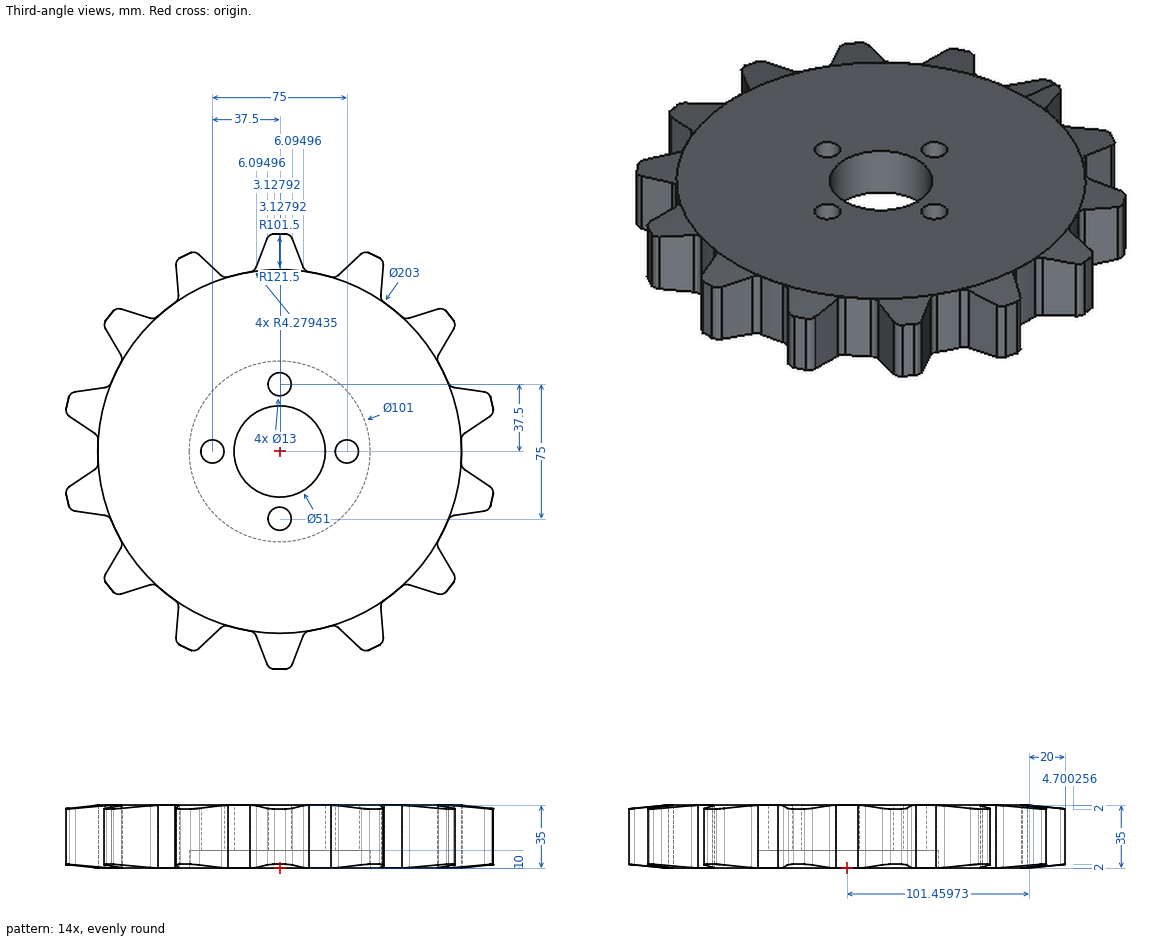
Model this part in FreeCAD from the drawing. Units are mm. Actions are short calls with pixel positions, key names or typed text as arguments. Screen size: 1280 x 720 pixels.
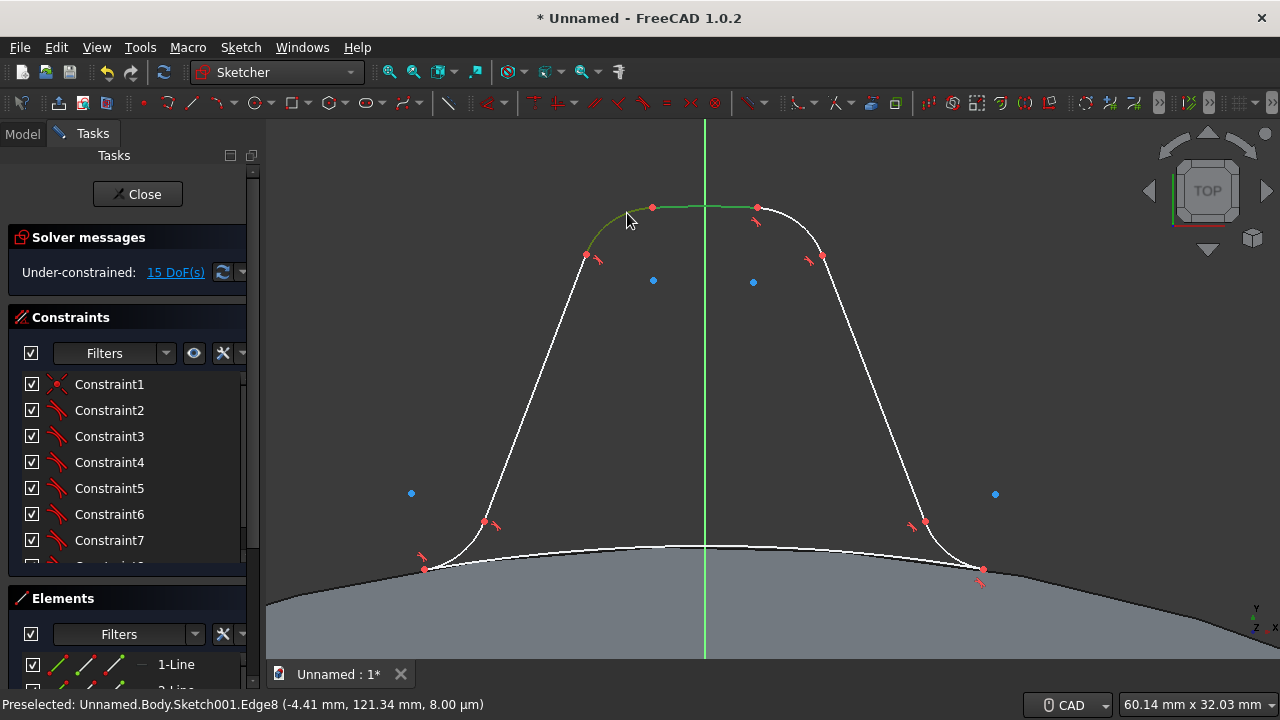
click(644, 104)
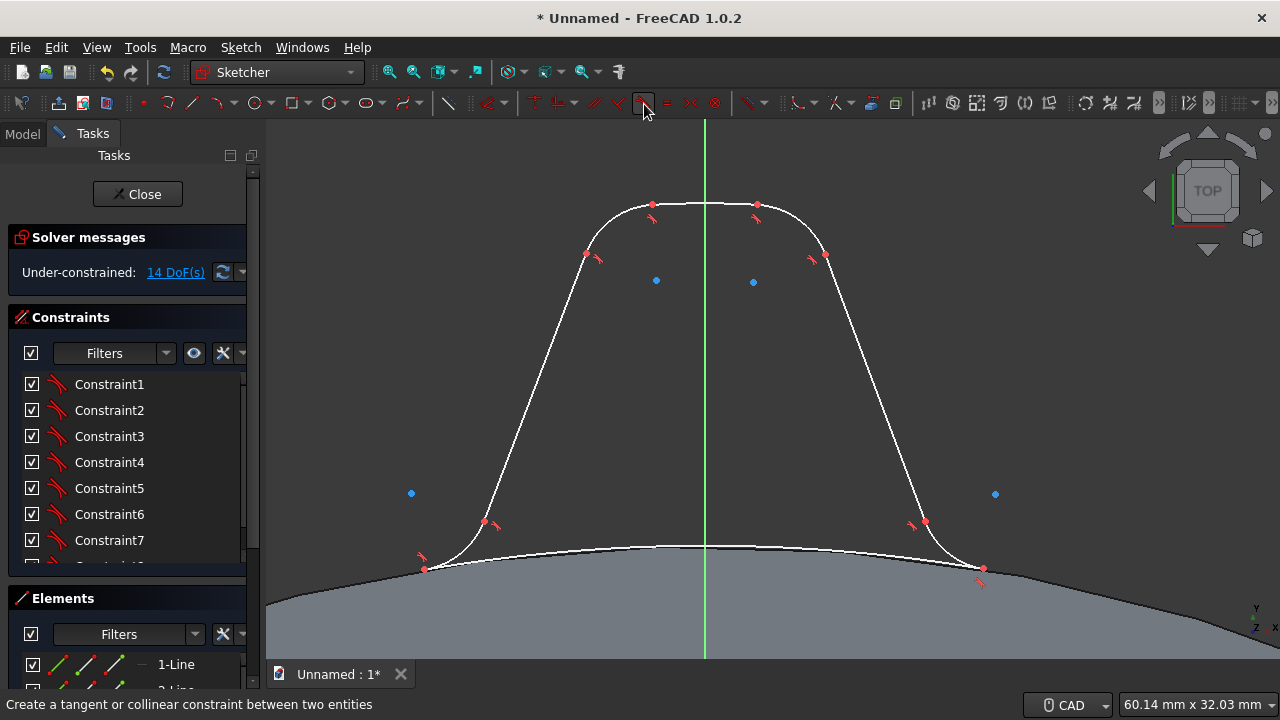
click(816, 549)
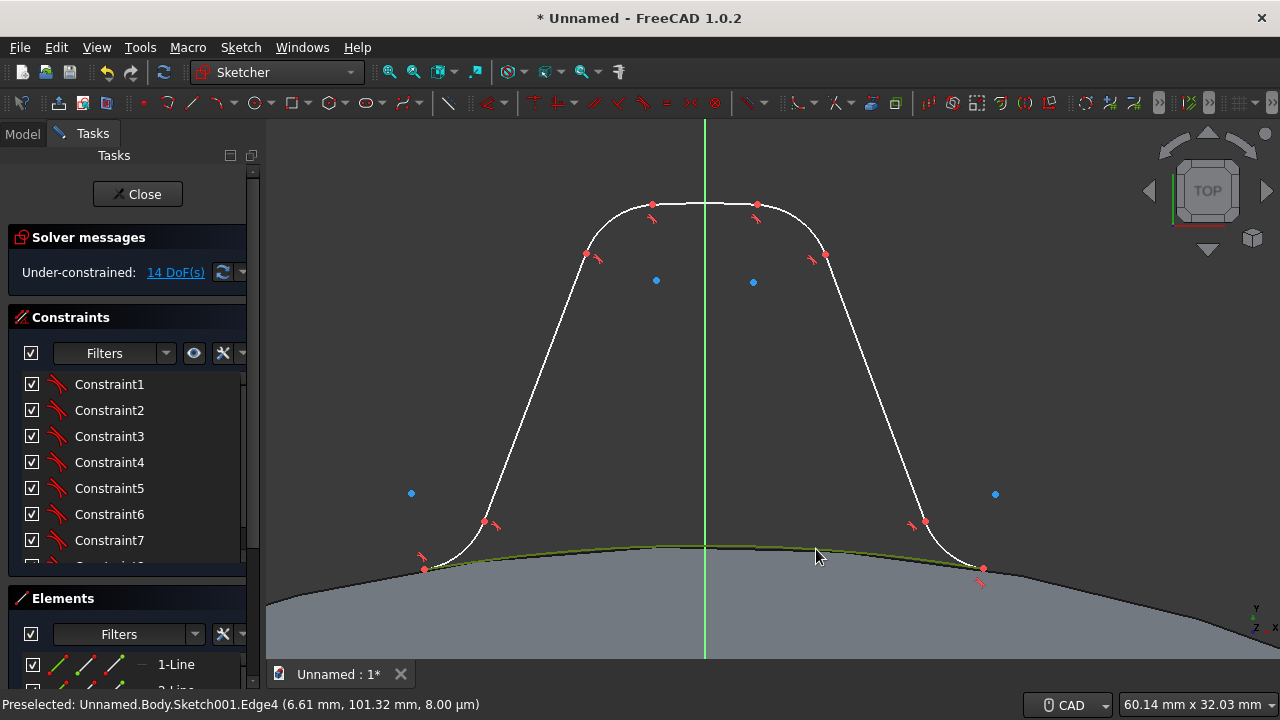
click(726, 204)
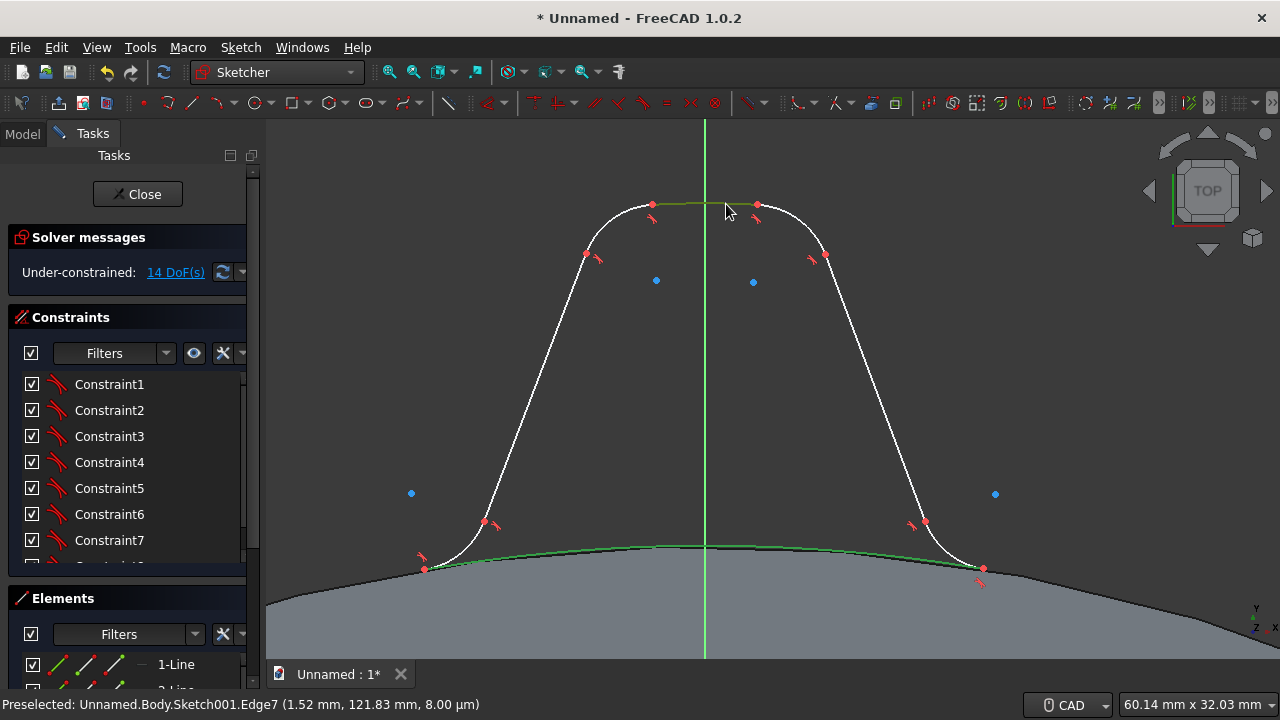
click(534, 104)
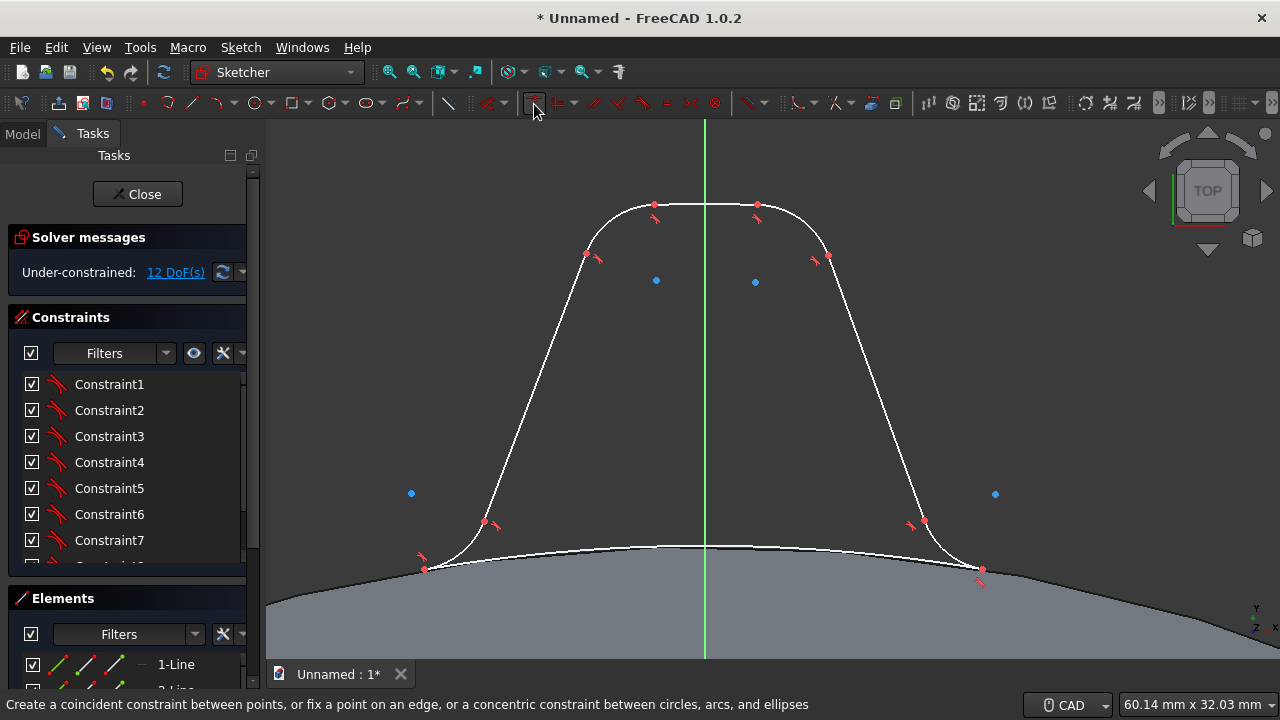
scroll(704, 224, down, 9)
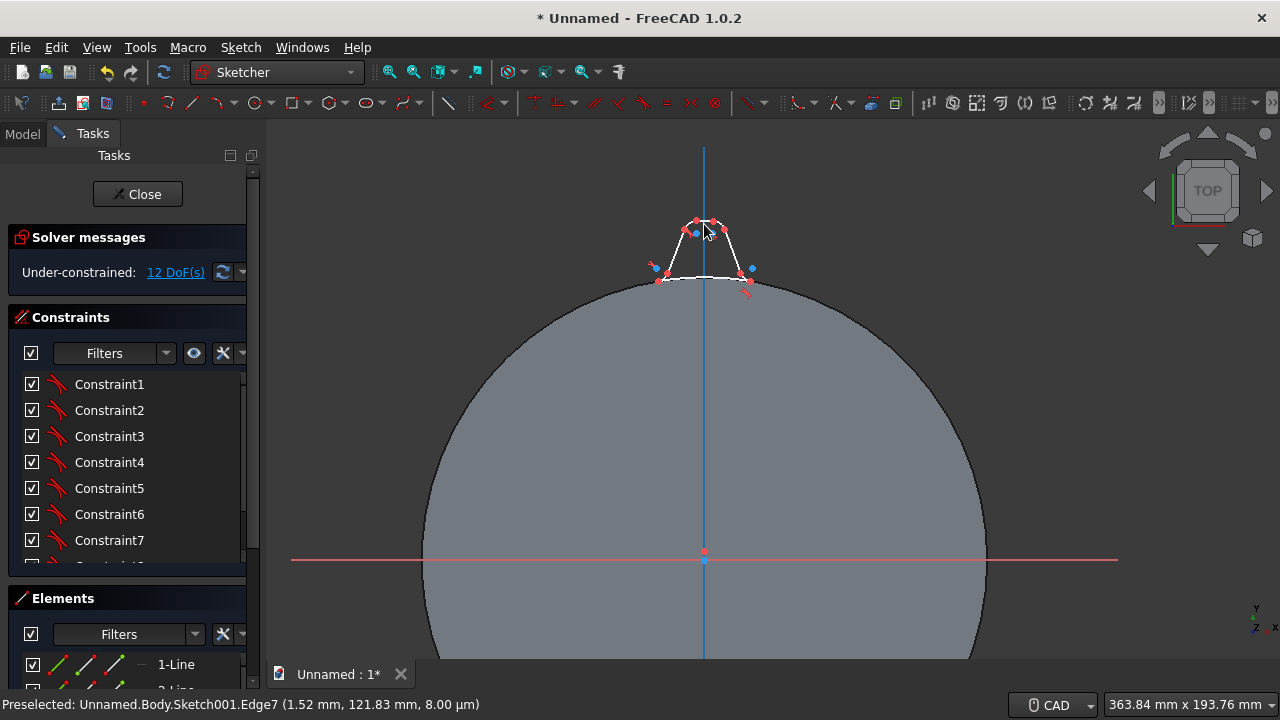
scroll(704, 556, up, 6)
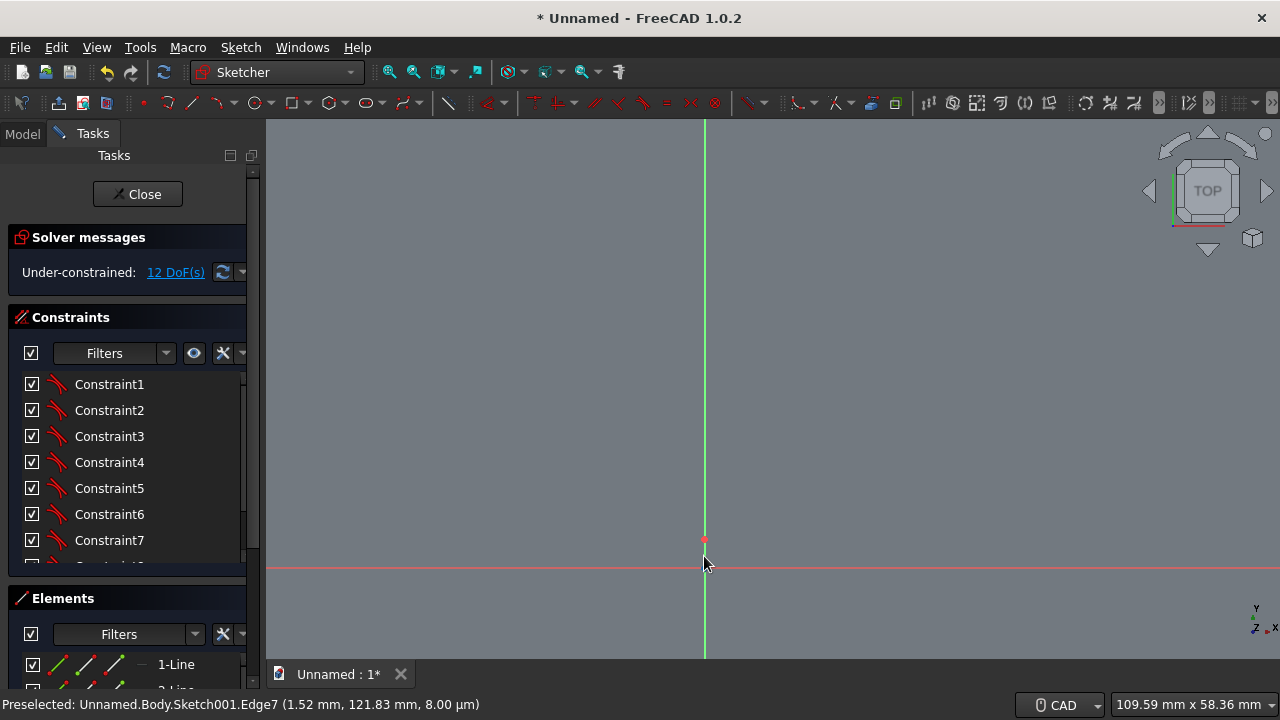
drag(695, 529, 715, 578)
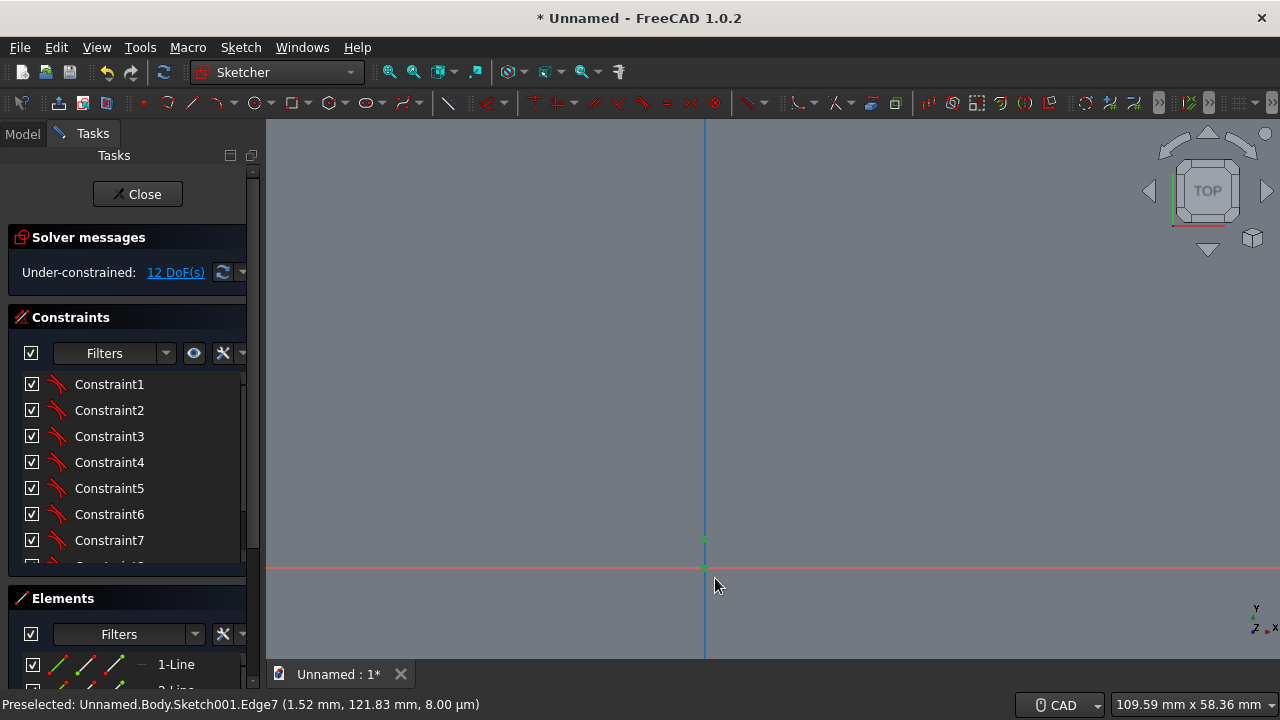
click(534, 104)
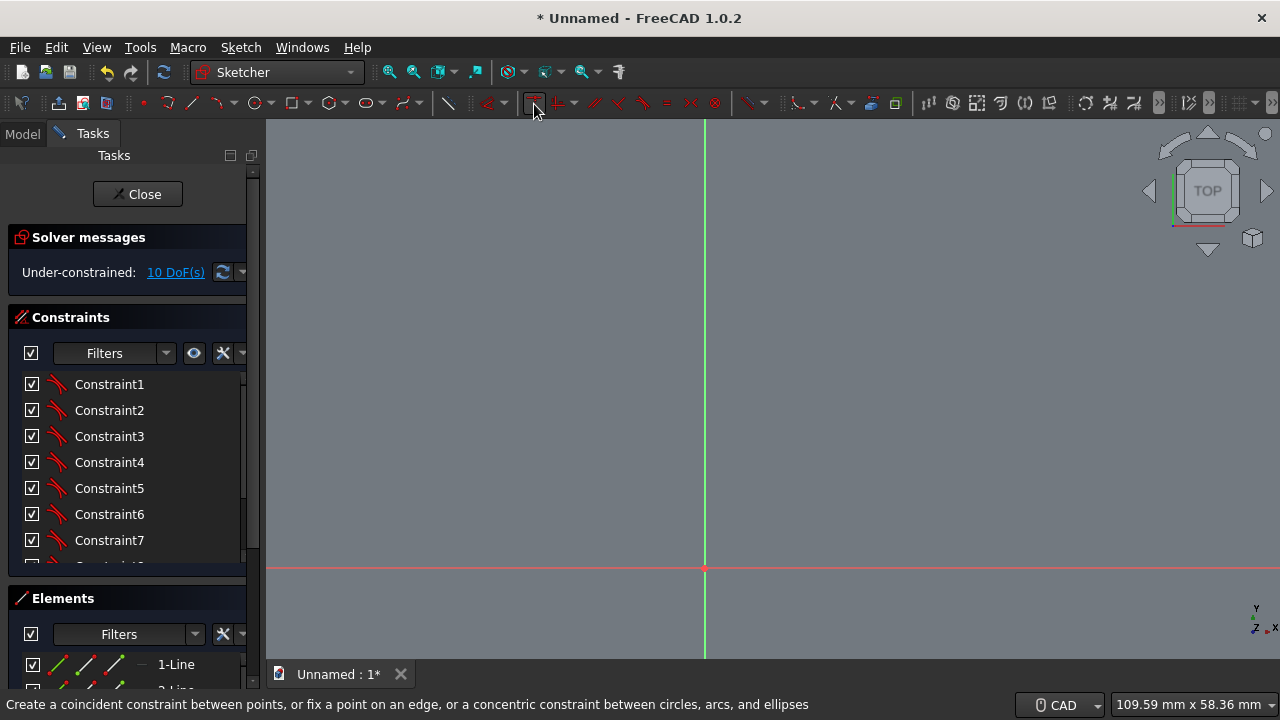
scroll(704, 389, down, 5)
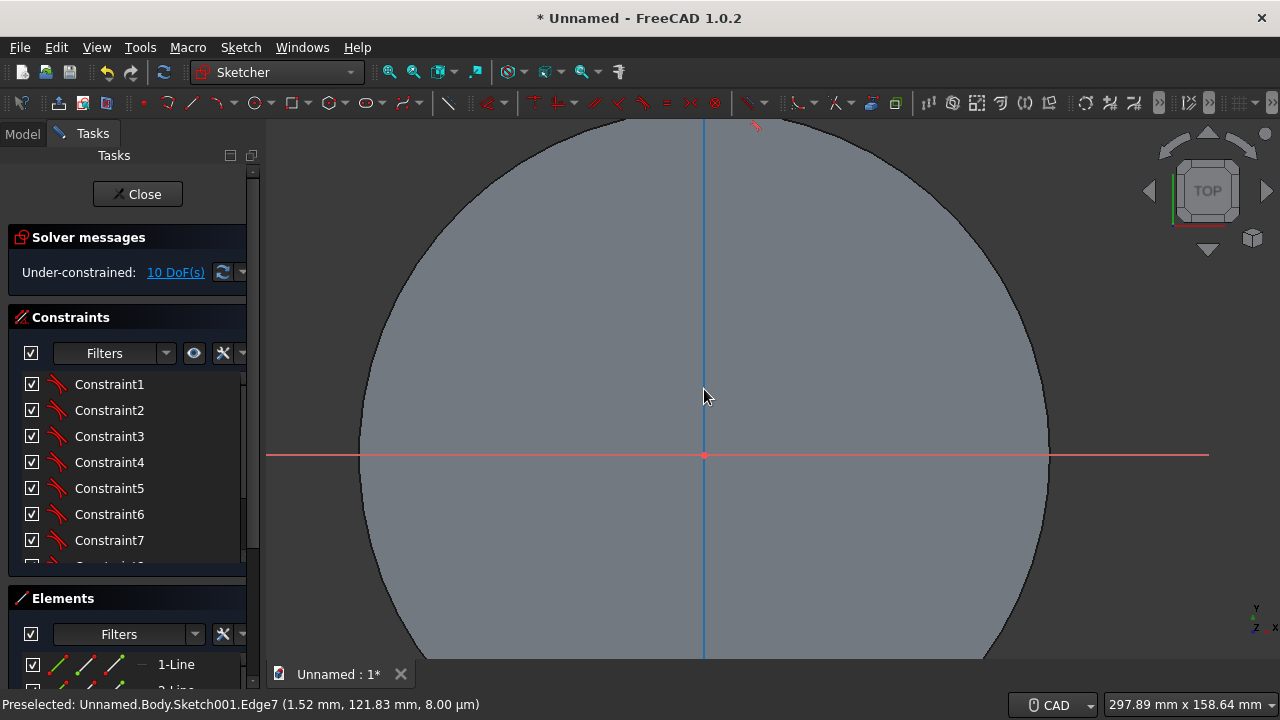
scroll(704, 389, down, 5)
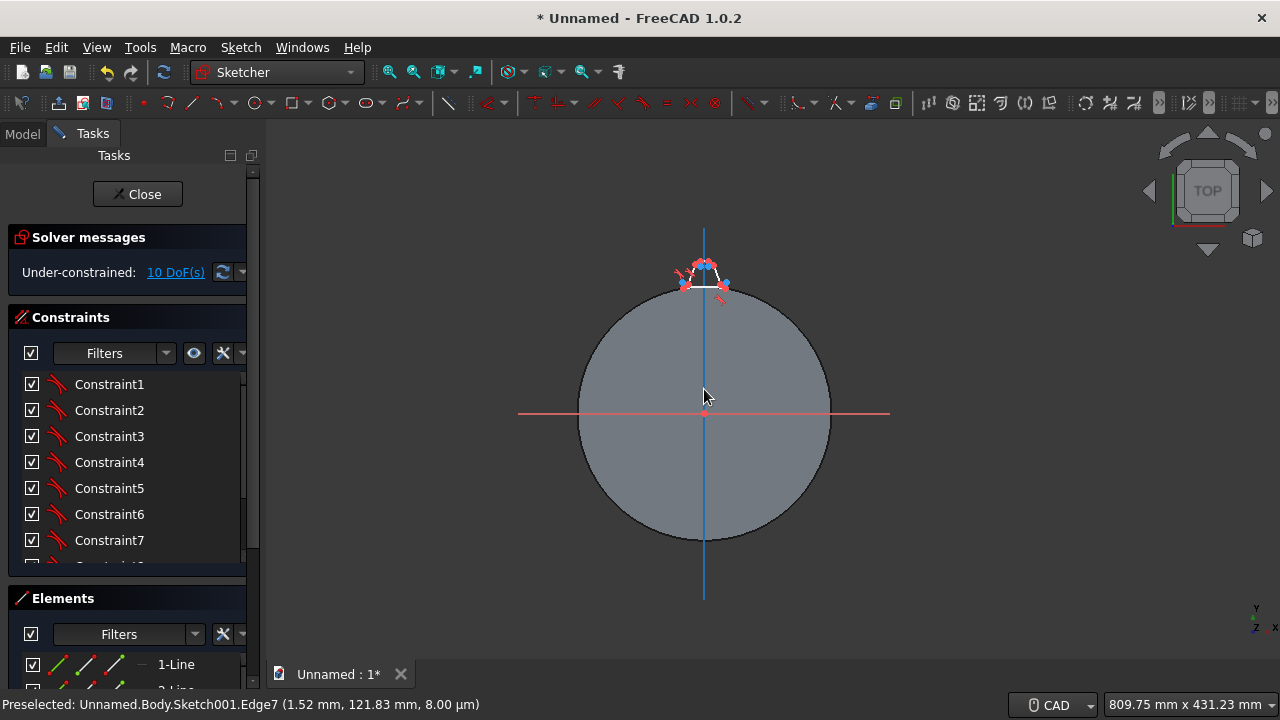
scroll(704, 266, up, 13)